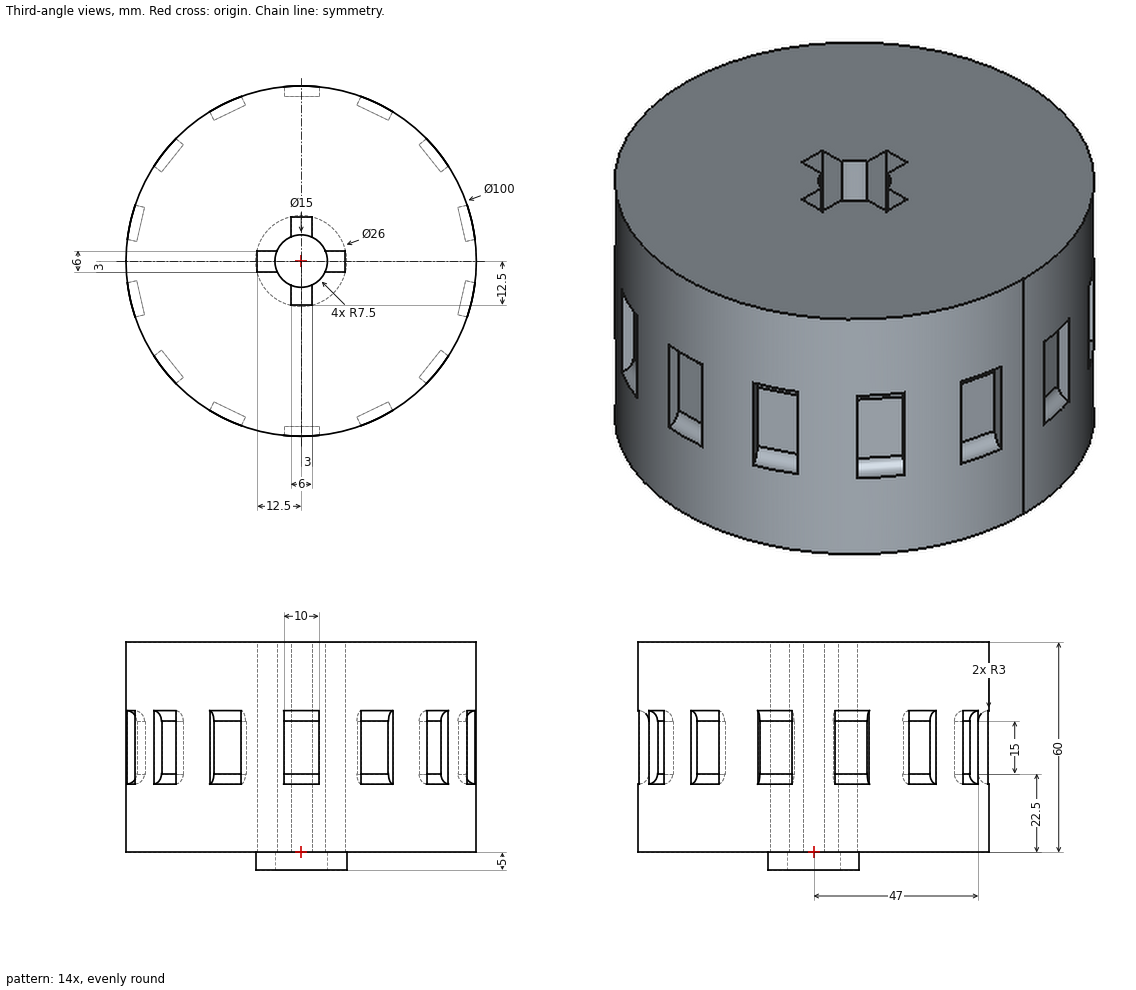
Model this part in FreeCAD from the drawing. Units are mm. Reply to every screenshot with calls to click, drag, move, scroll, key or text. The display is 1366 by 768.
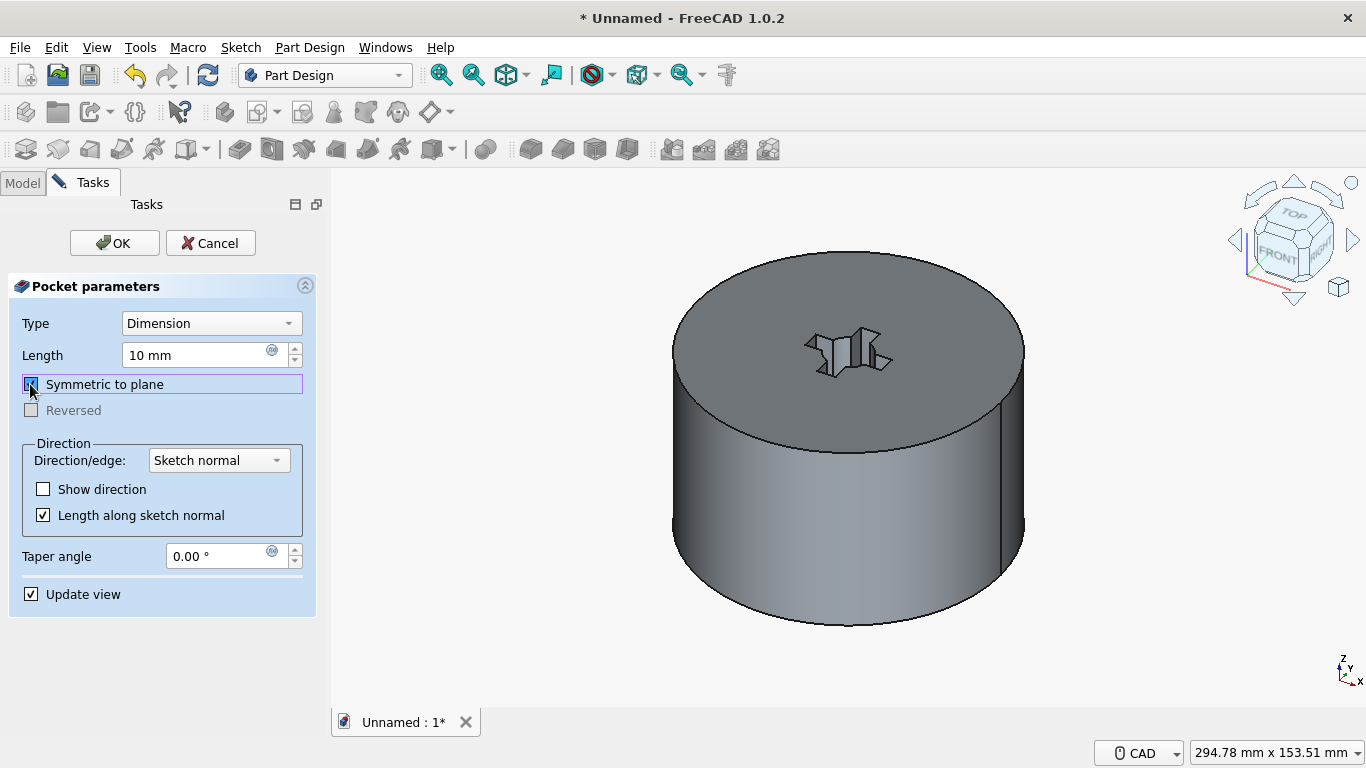
click(115, 243)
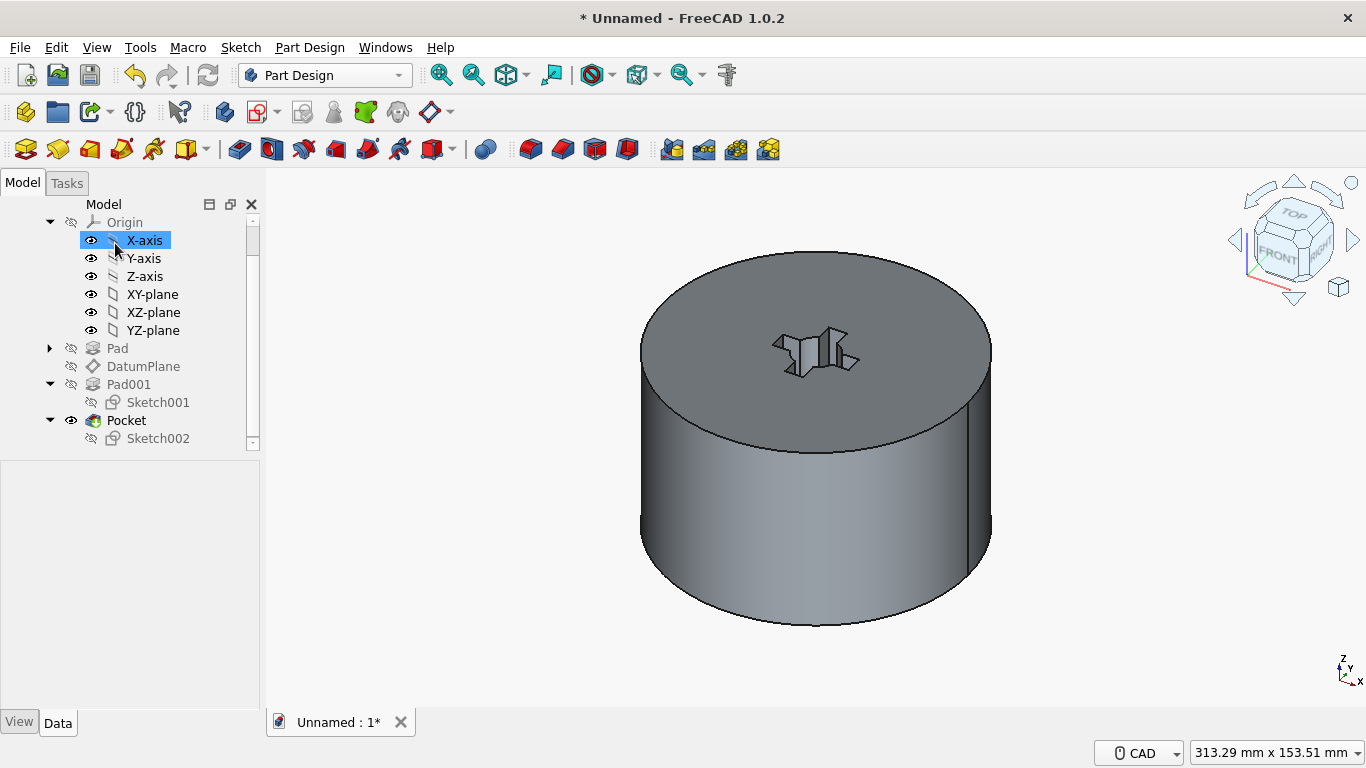
click(116, 420)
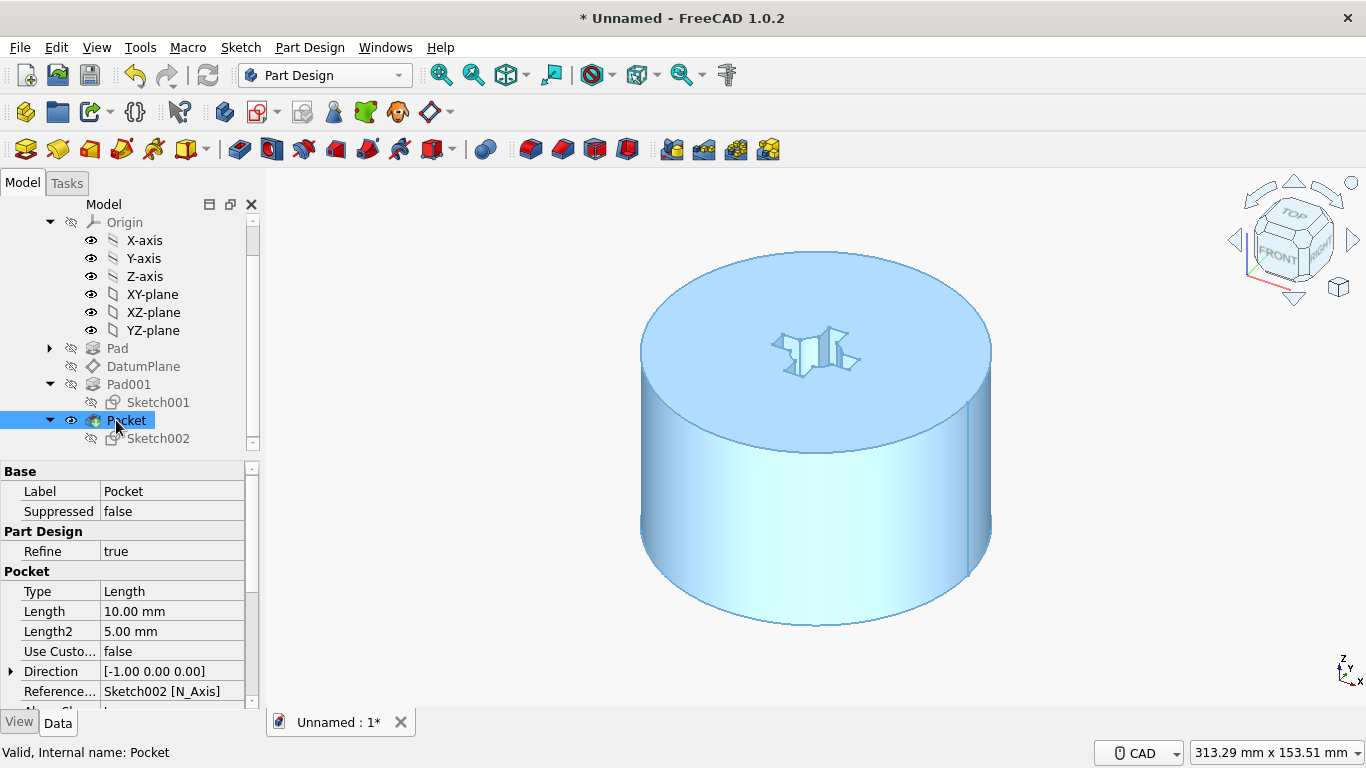
click(736, 150)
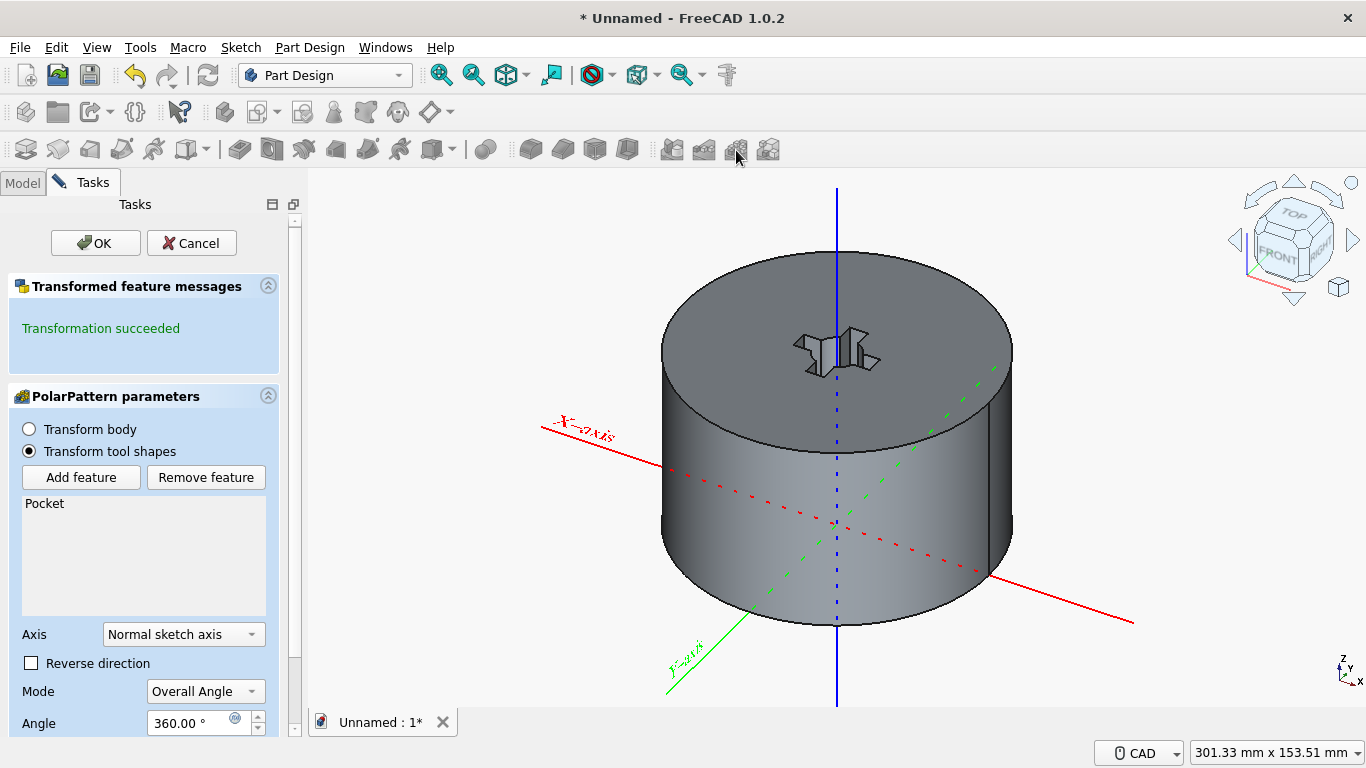
click(184, 634)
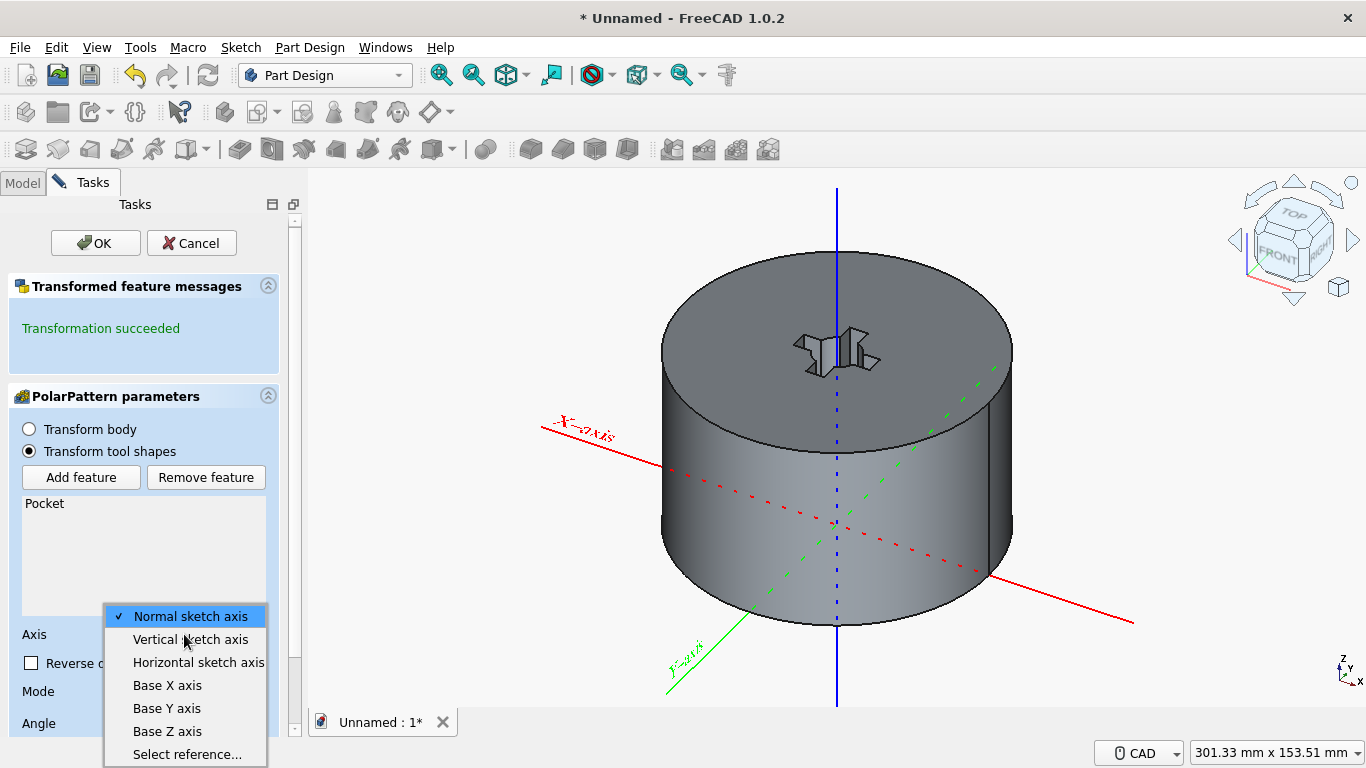
click(184, 732)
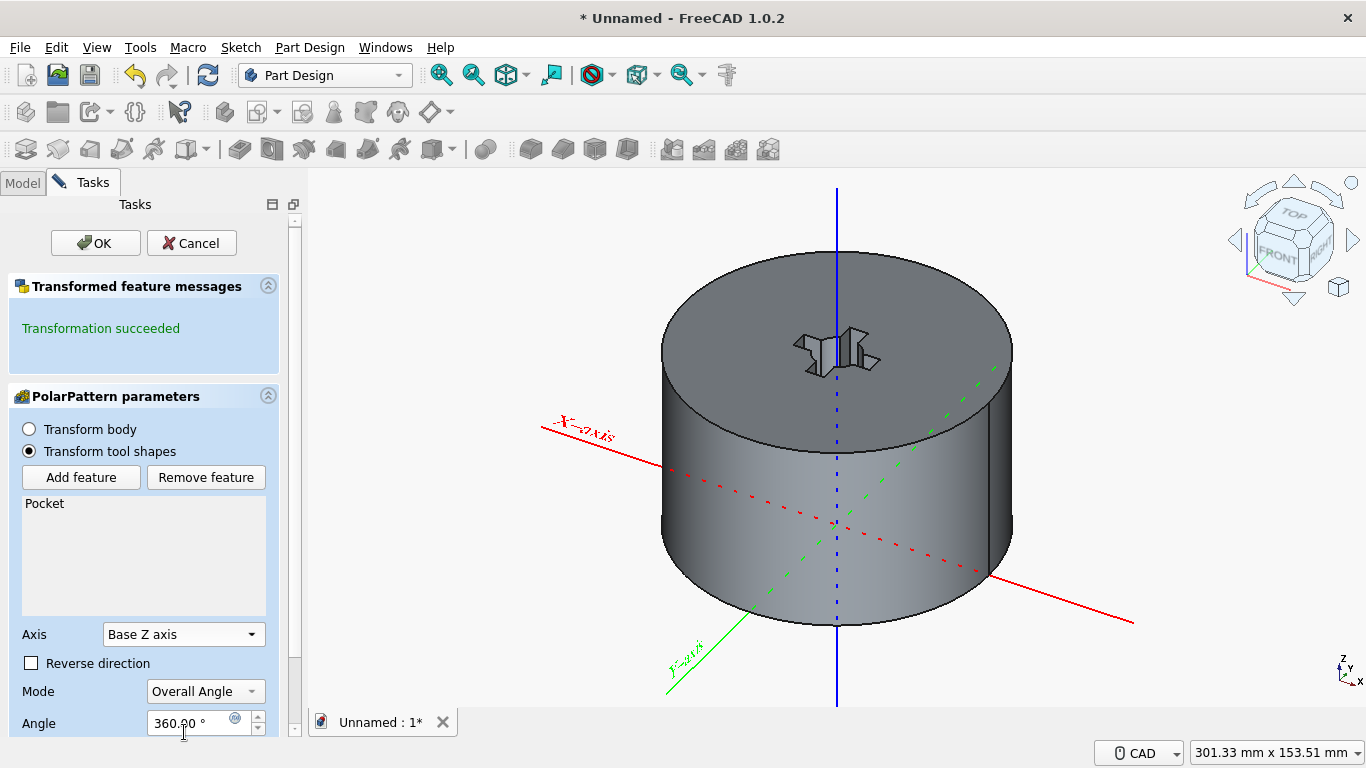
scroll(295, 475, down, 2)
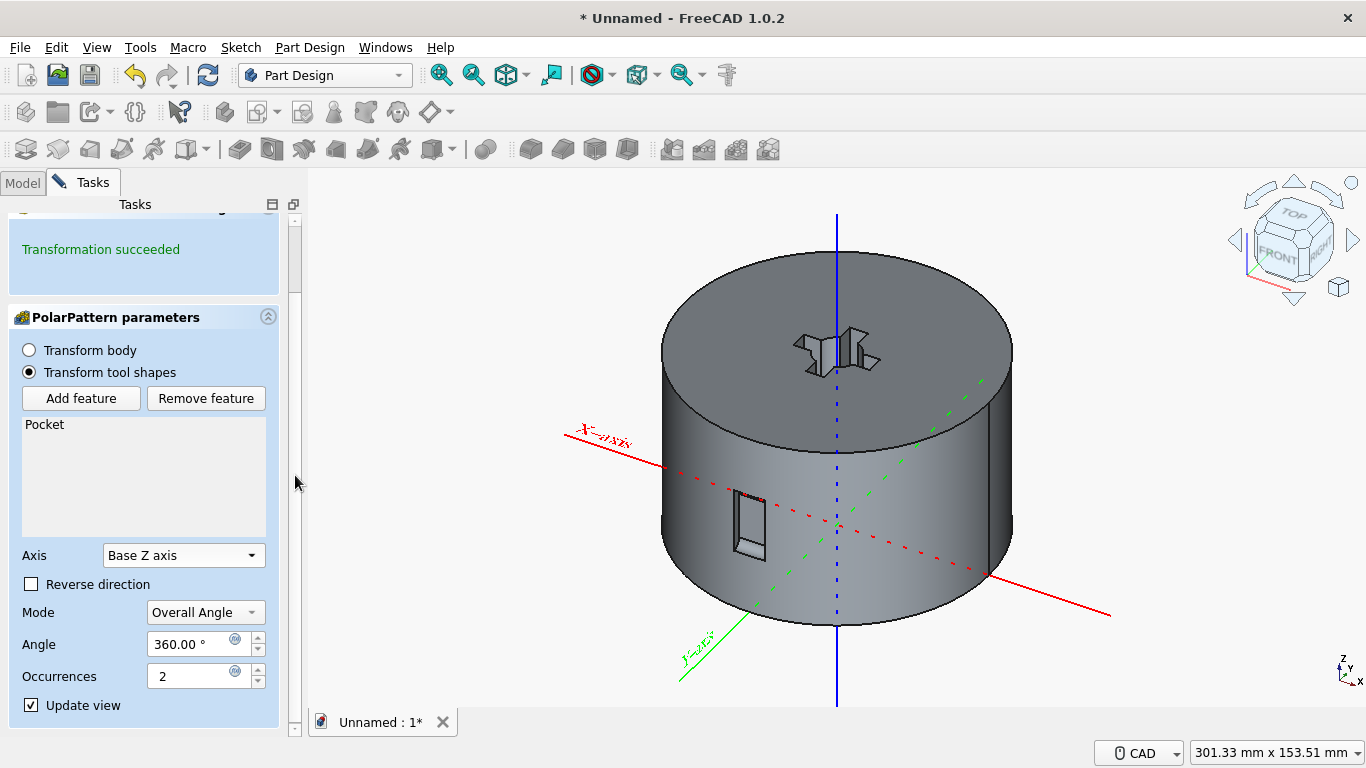
triple_click(198, 676)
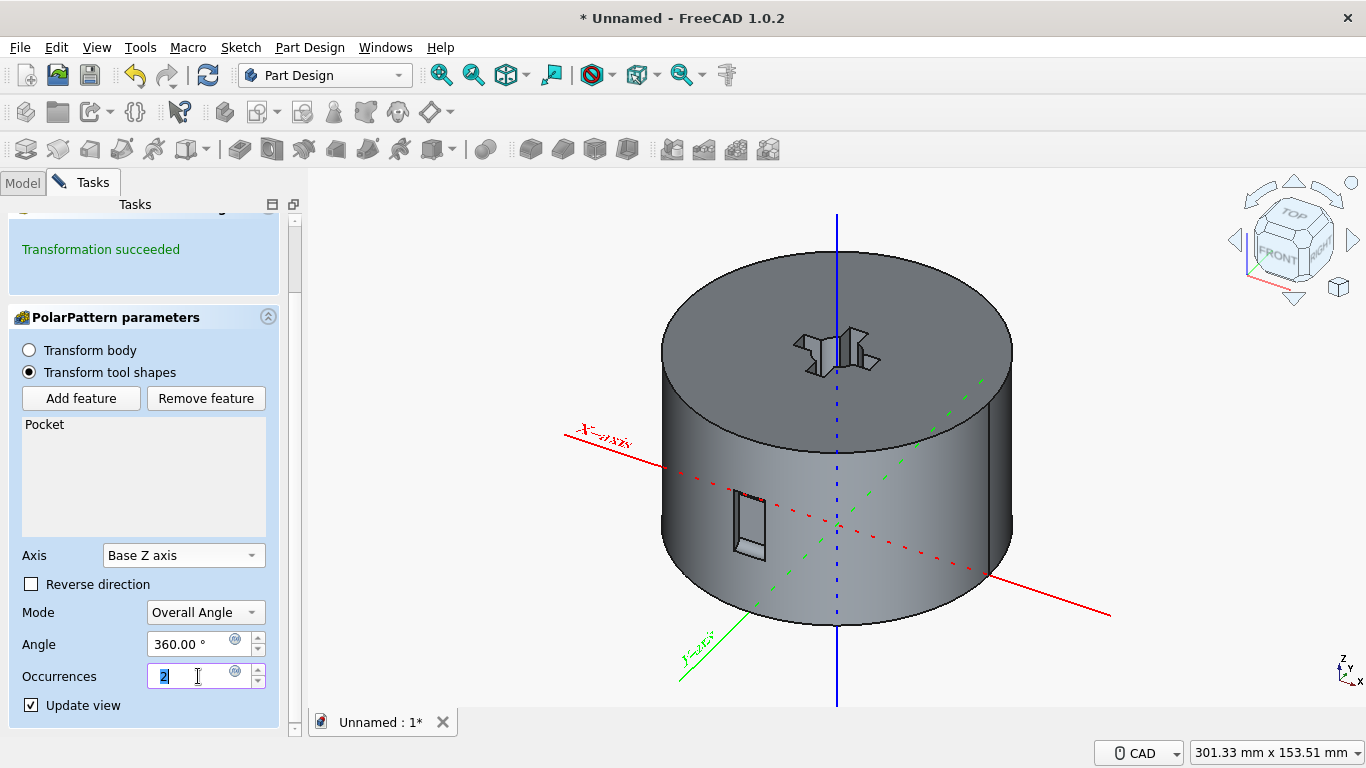
text(14)
key(Tab)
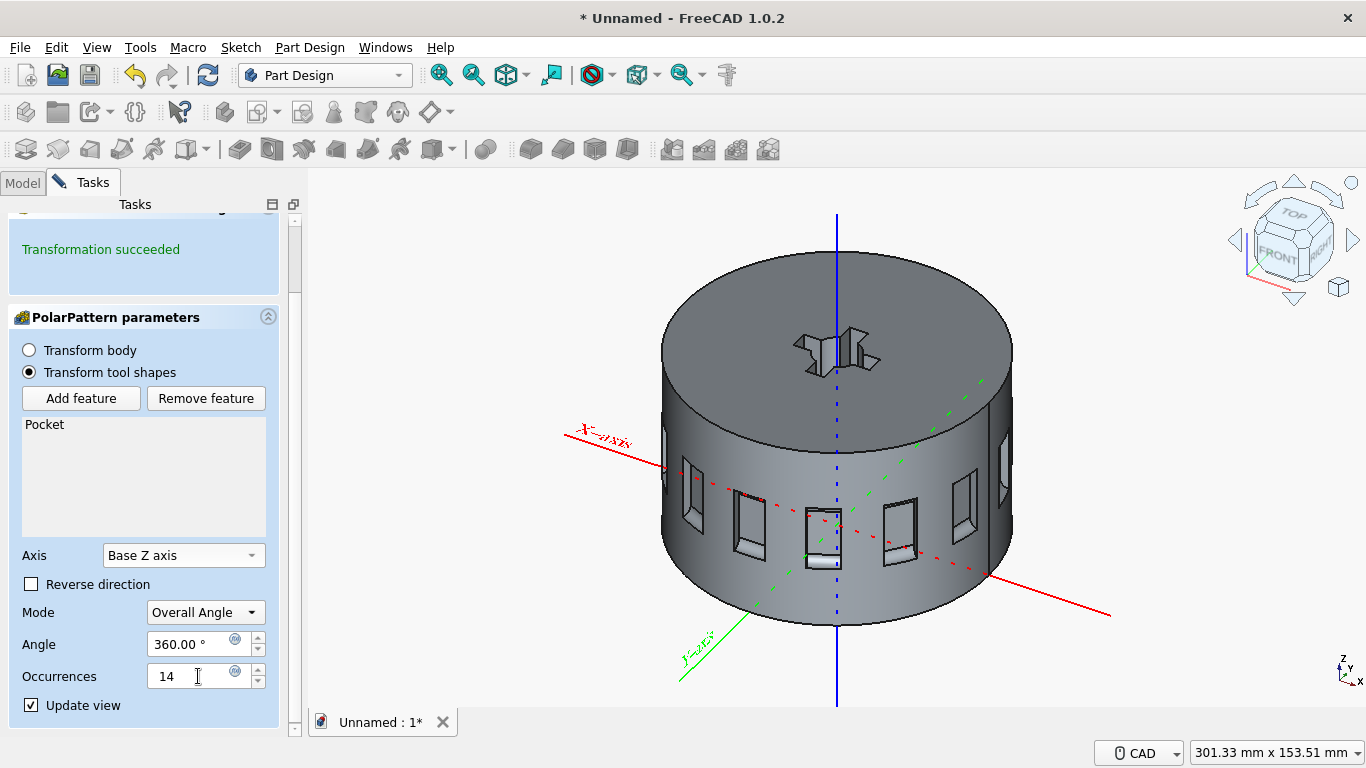
scroll(295, 475, up, 3)